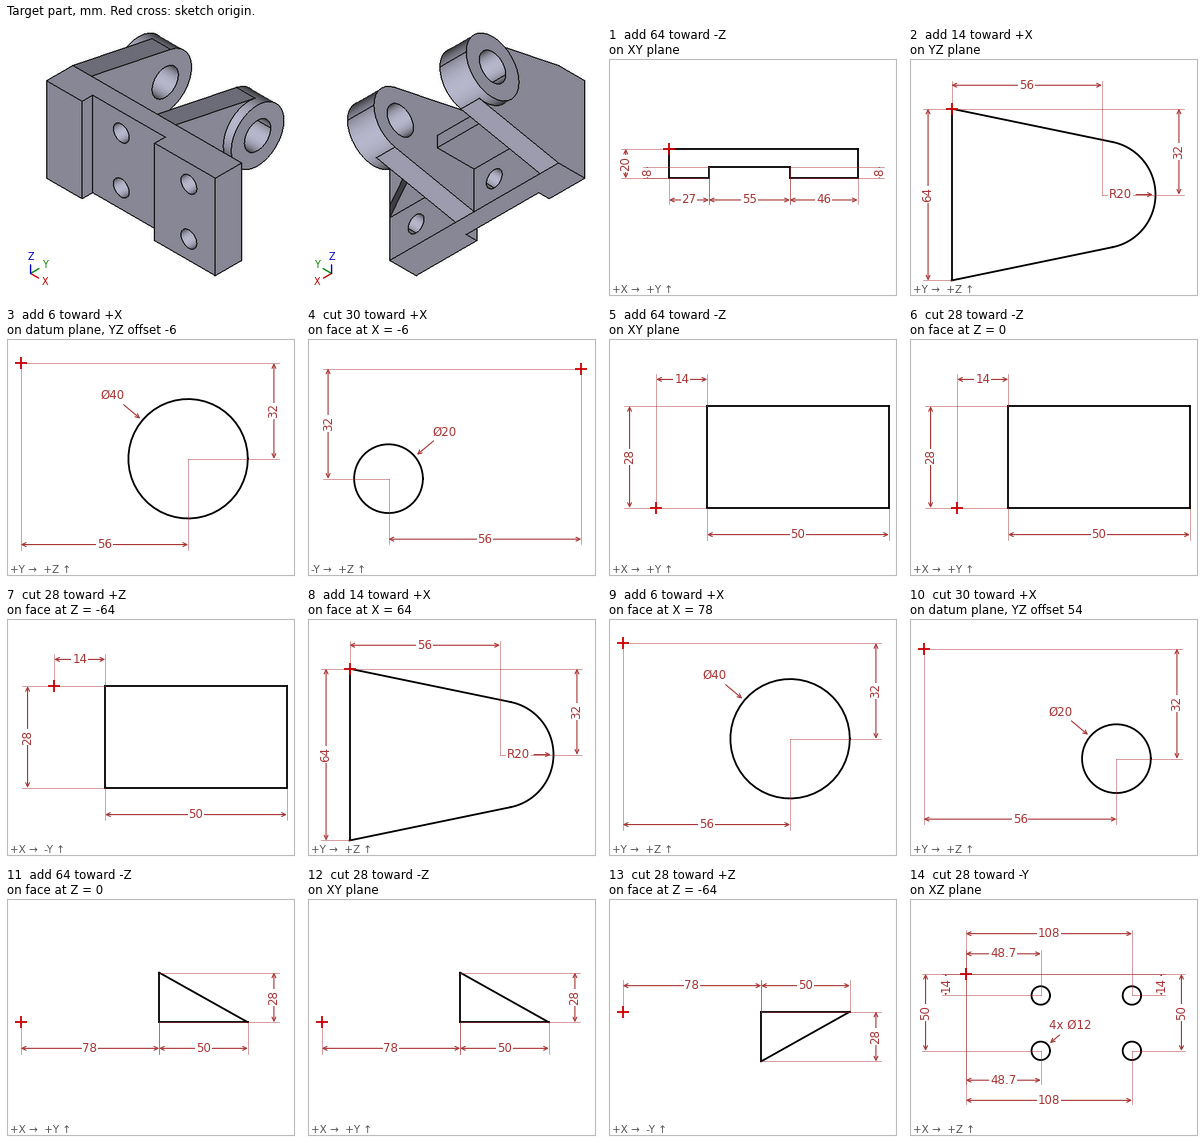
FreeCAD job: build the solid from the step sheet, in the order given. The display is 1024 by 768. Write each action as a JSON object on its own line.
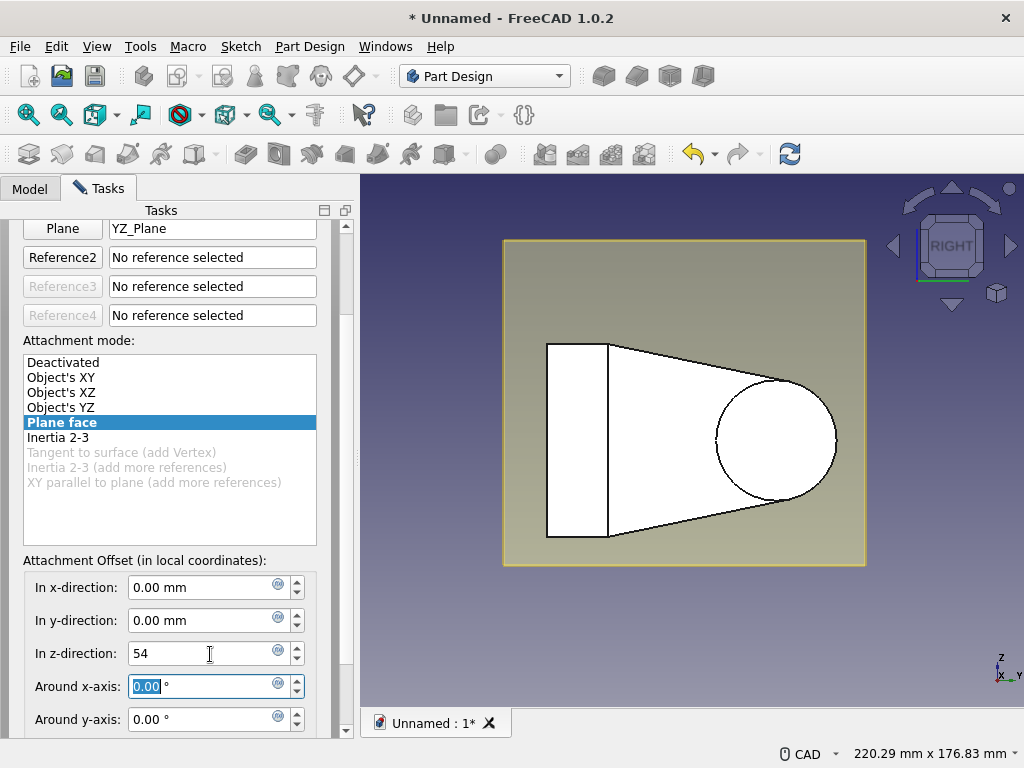
{"action": "scroll", "coordinate": [346, 479], "scroll_direction": "up", "scroll_amount": 3}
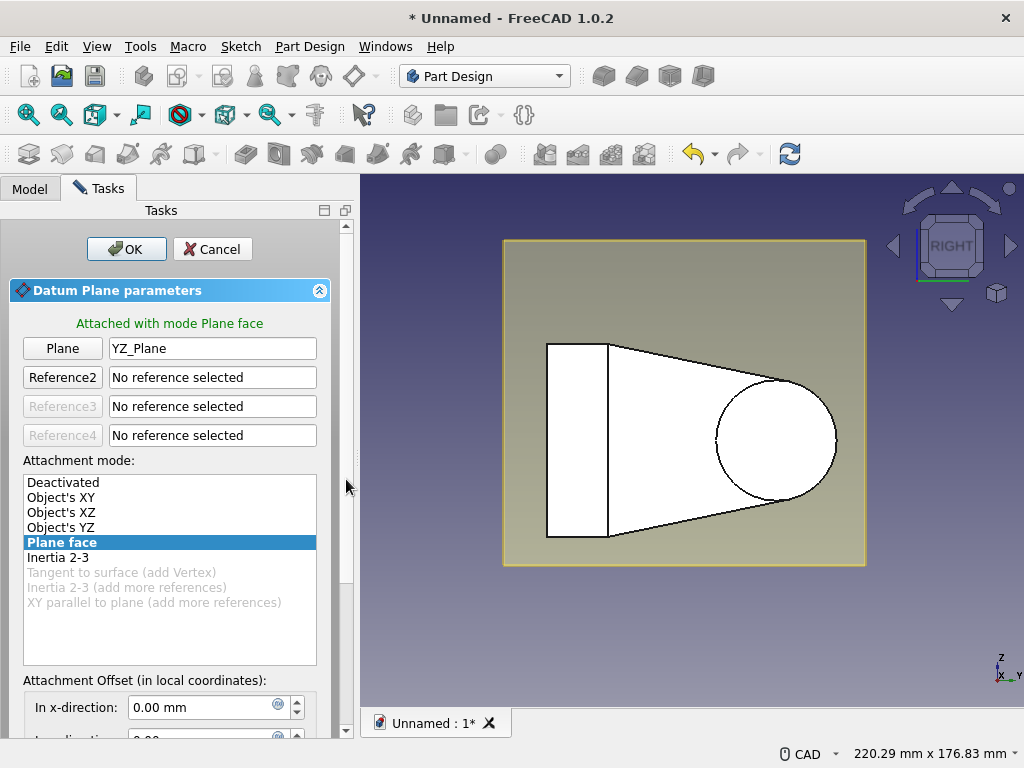
{"action": "left_click", "coordinate": [127, 249]}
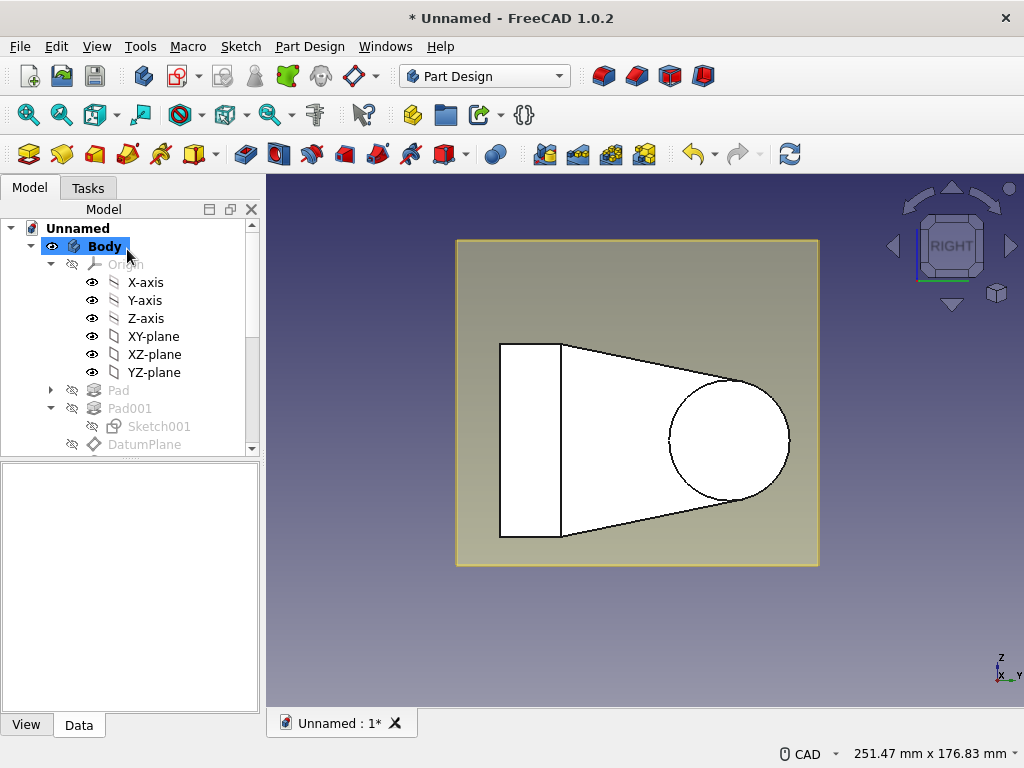
{"action": "scroll", "coordinate": [101, 332], "scroll_direction": "down", "scroll_amount": 3}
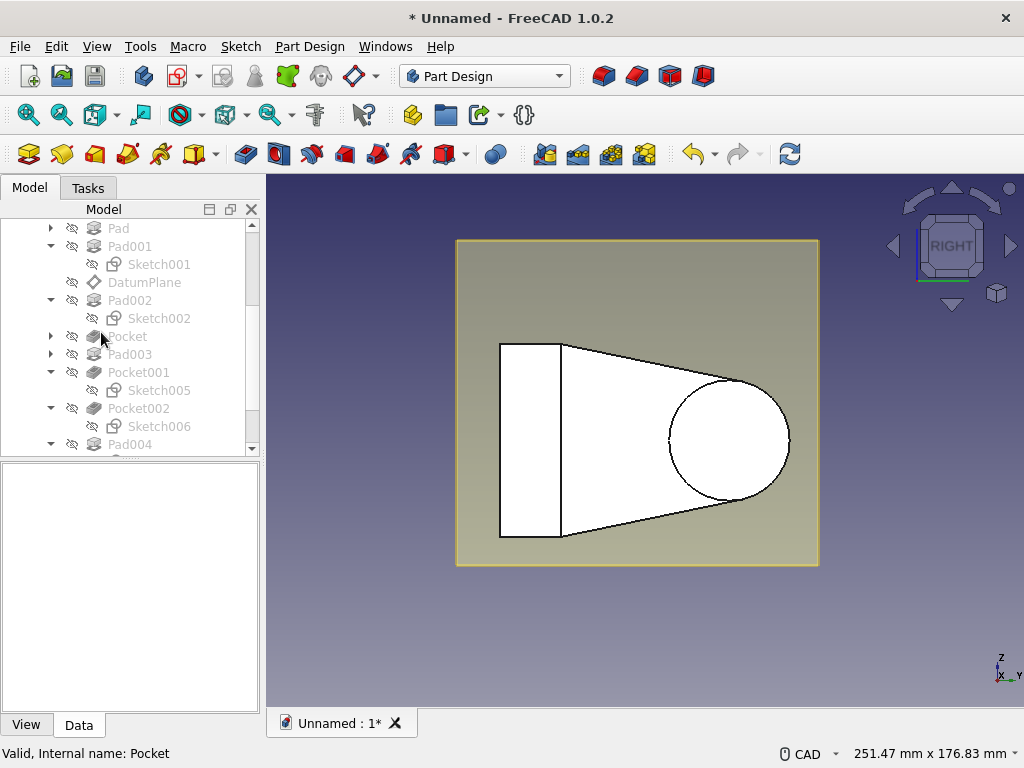
{"action": "scroll", "coordinate": [141, 332], "scroll_direction": "up", "scroll_amount": 15}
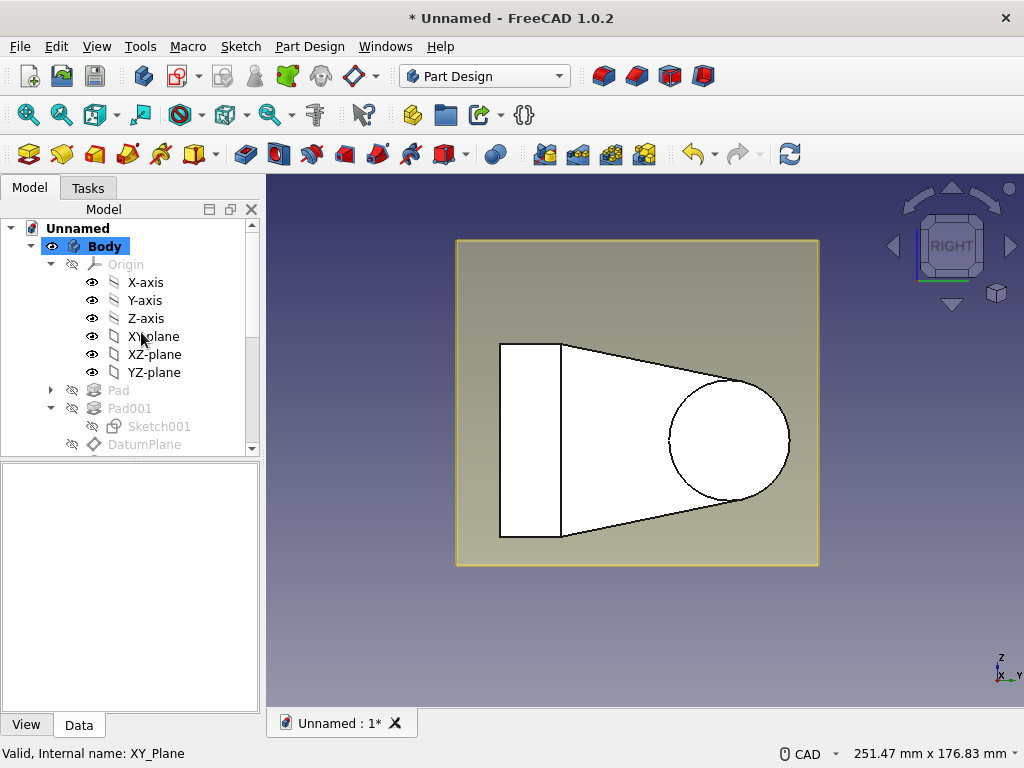
{"action": "scroll", "coordinate": [101, 332], "scroll_direction": "down", "scroll_amount": 6}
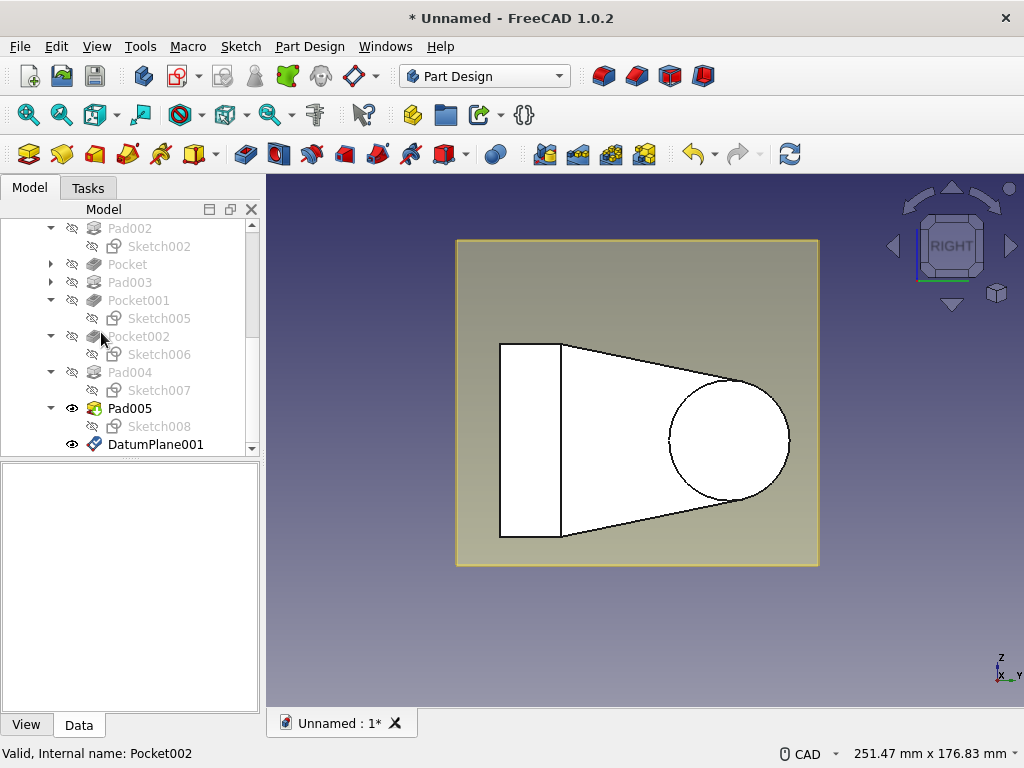
{"action": "left_click", "coordinate": [117, 444]}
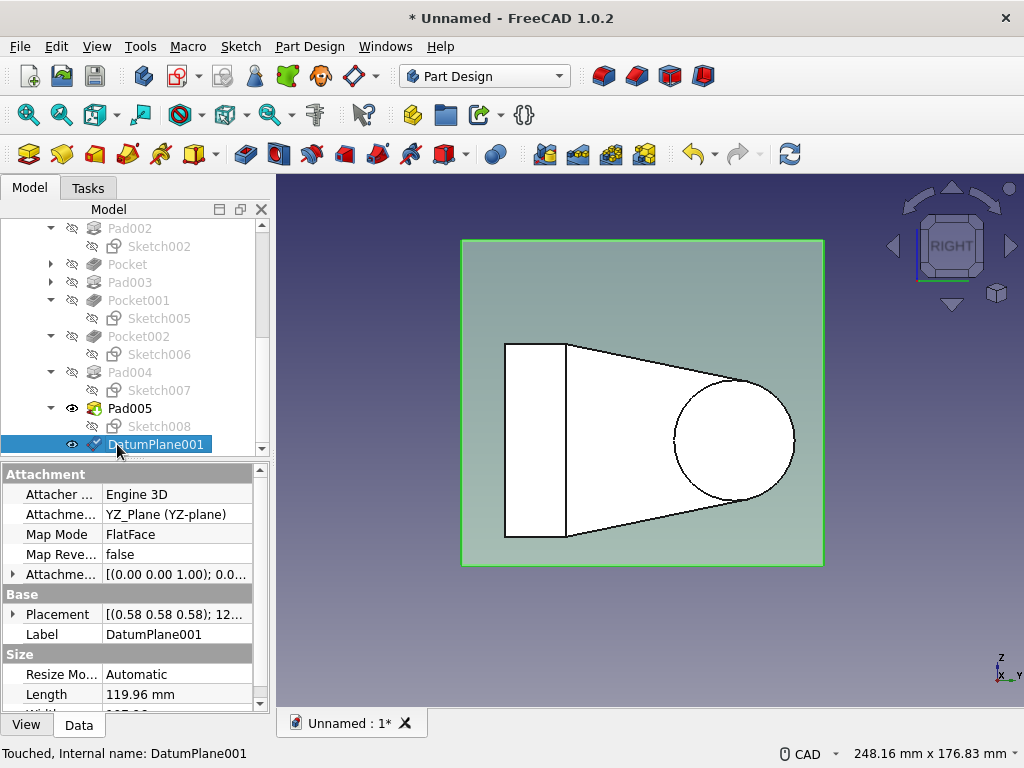
{"action": "left_click", "coordinate": [176, 76]}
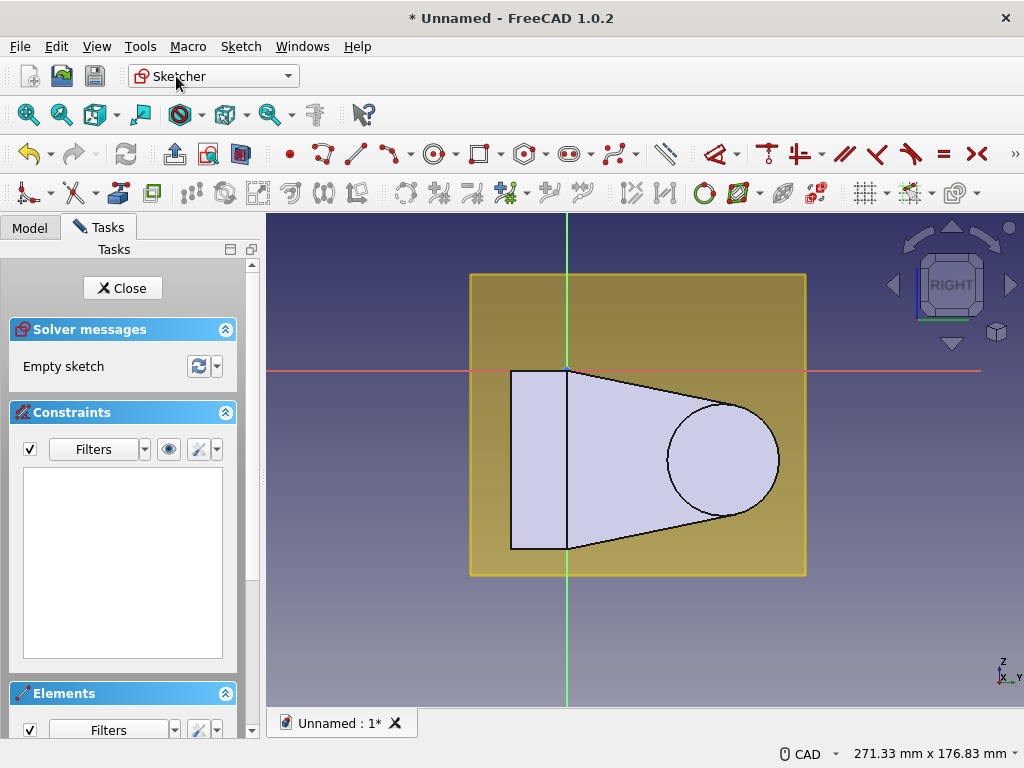
{"action": "left_click", "coordinate": [241, 154]}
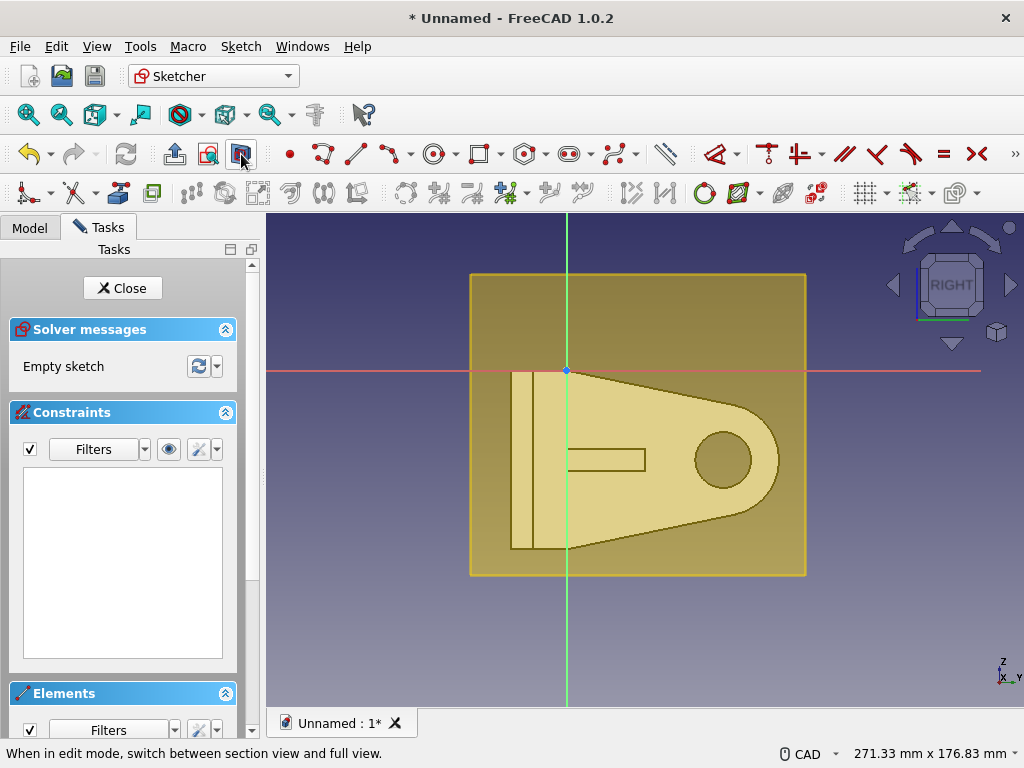
{"action": "scroll", "coordinate": [752, 460], "scroll_direction": "up", "scroll_amount": 9}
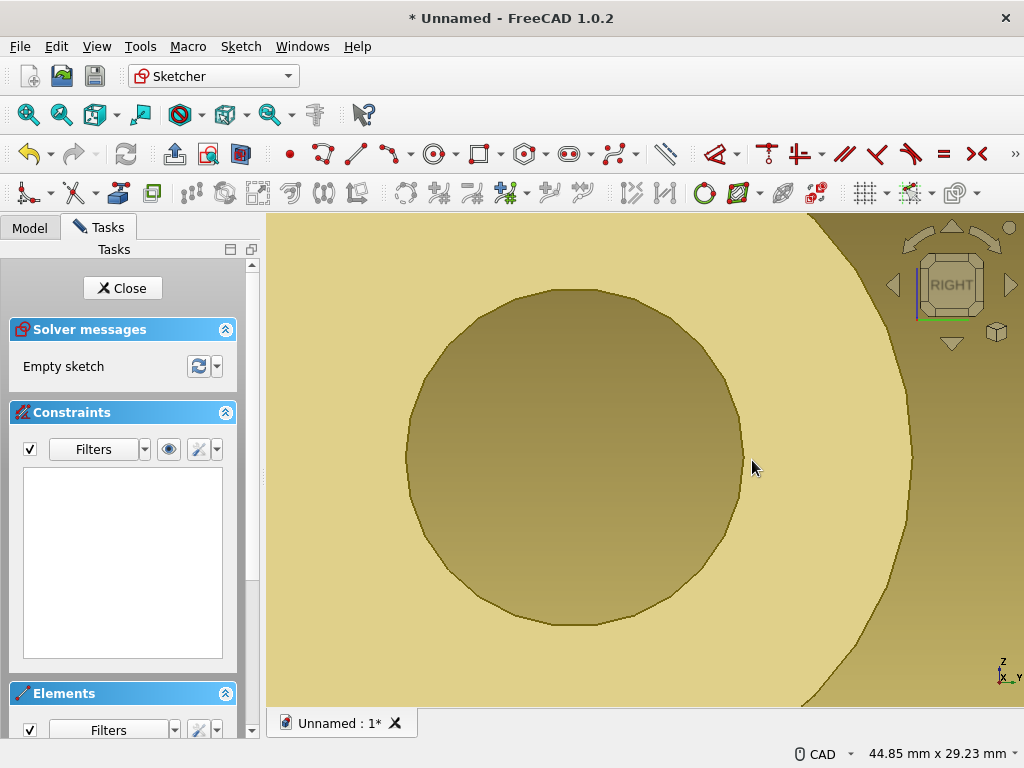
{"action": "left_click", "coordinate": [434, 154]}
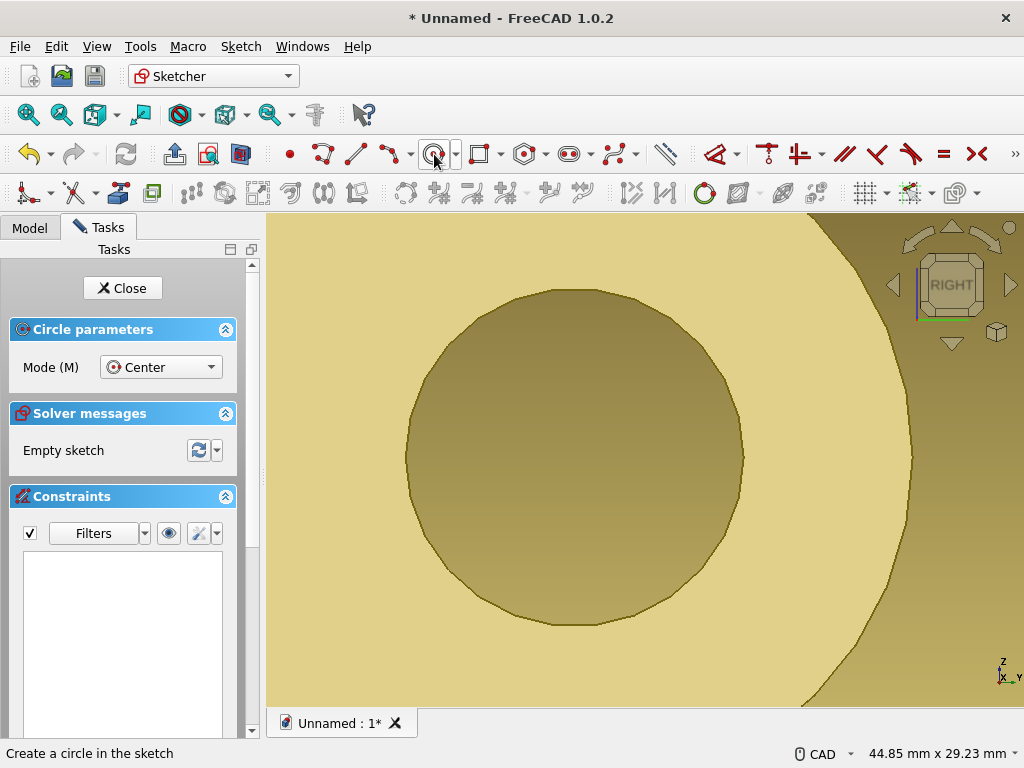
{"action": "left_click", "coordinate": [575, 457]}
{"action": "left_click", "coordinate": [694, 338]}
{"action": "key", "text": "Escape"}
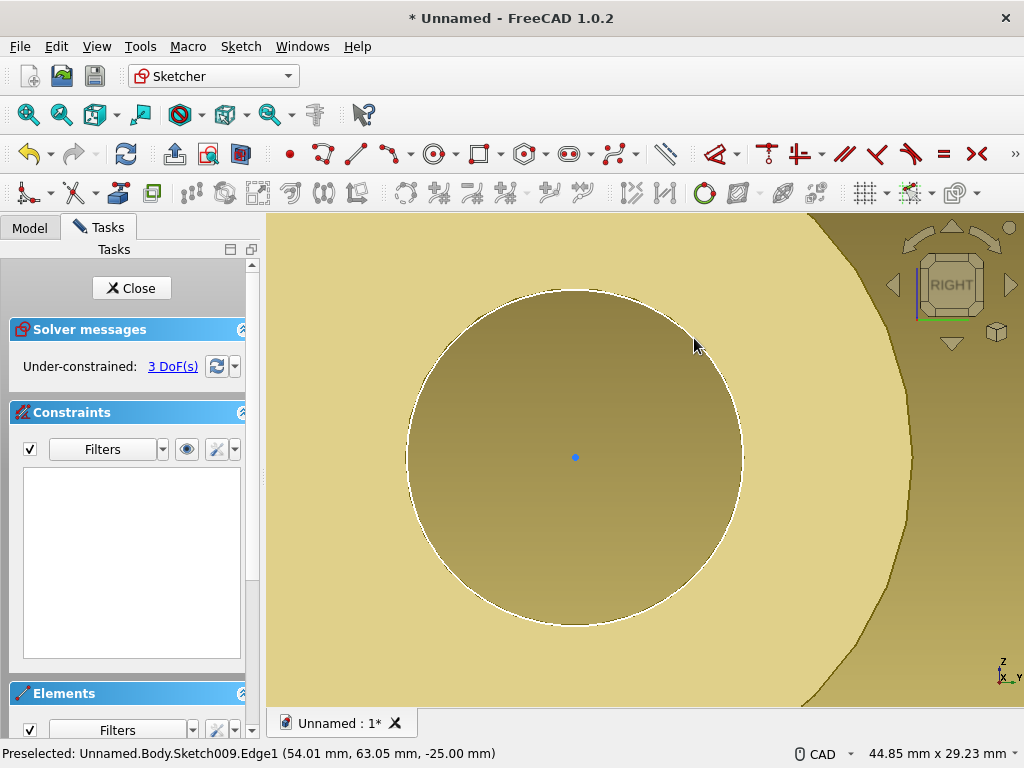
{"action": "left_click", "coordinate": [714, 154]}